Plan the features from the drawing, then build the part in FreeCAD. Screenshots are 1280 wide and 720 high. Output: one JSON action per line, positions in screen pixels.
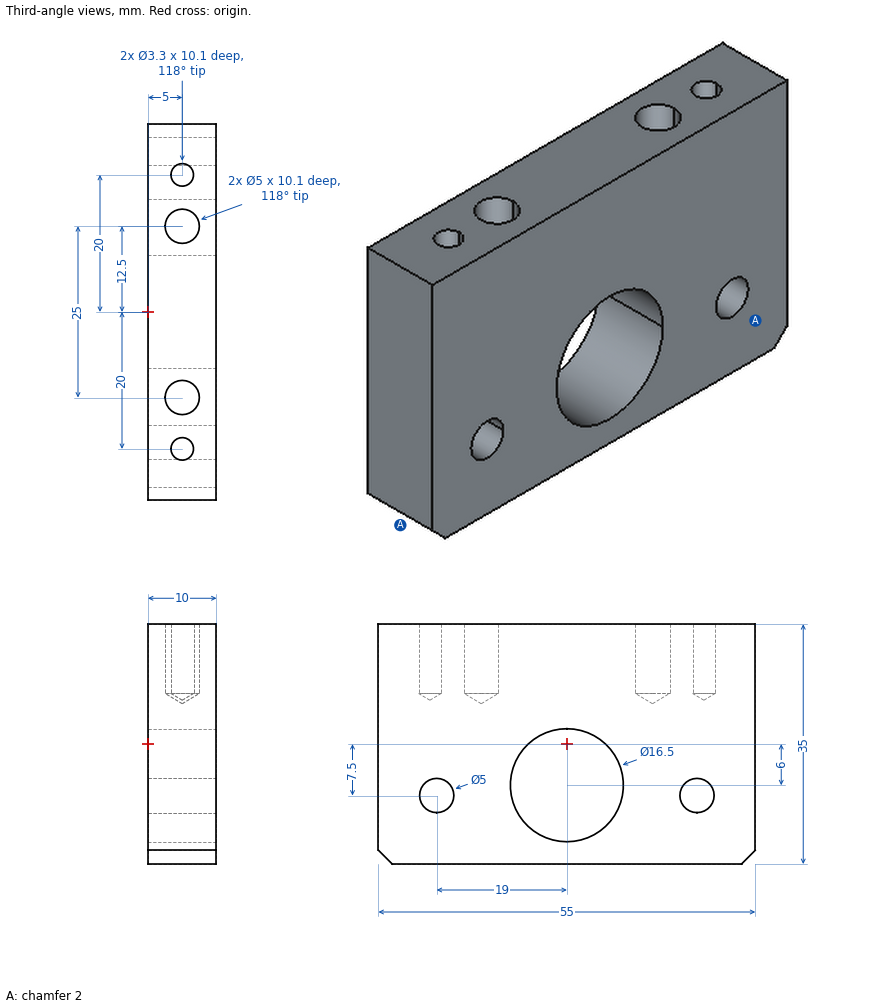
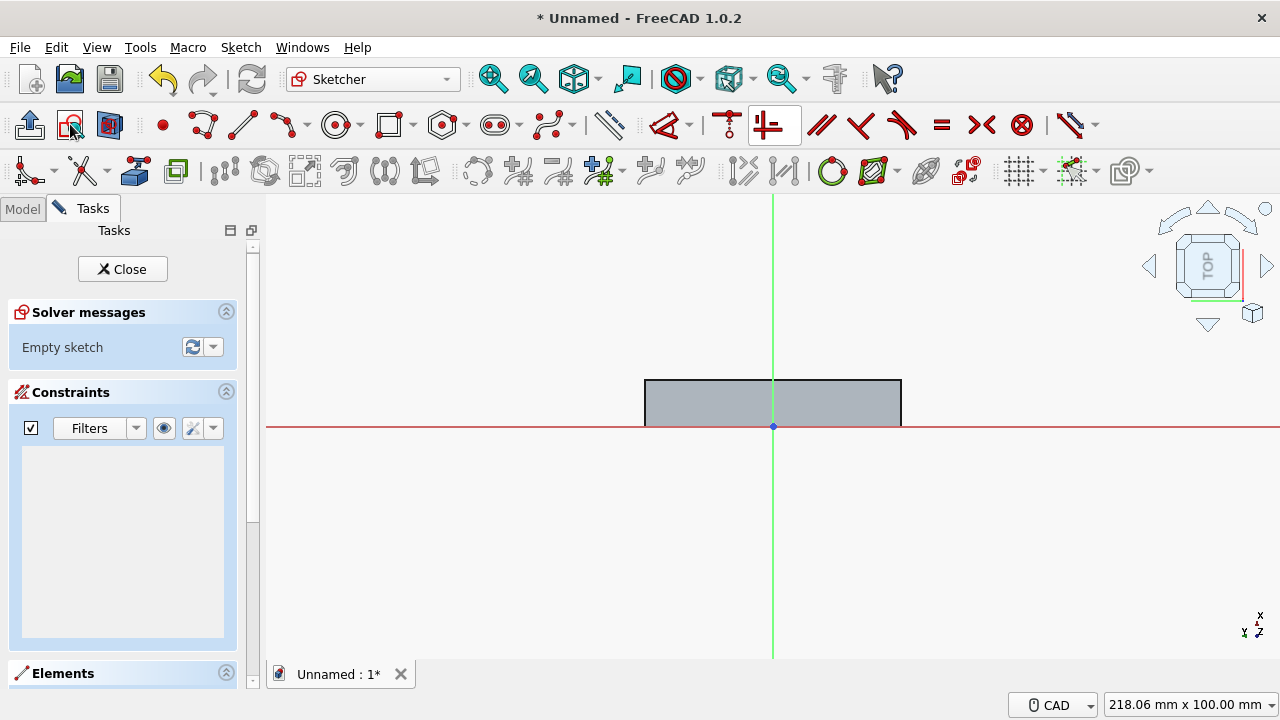
{"action": "scroll", "coordinate": [813, 402], "scroll_direction": "up", "scroll_amount": 5}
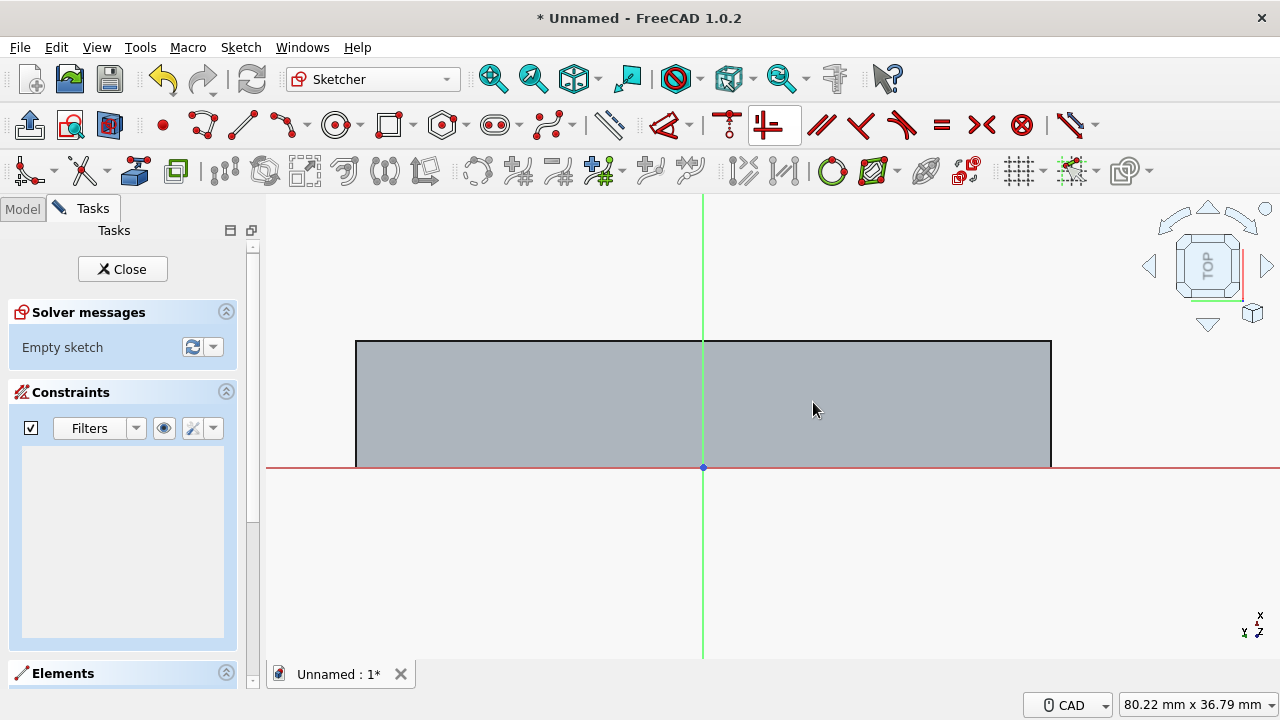
{"action": "left_click", "coordinate": [336, 126]}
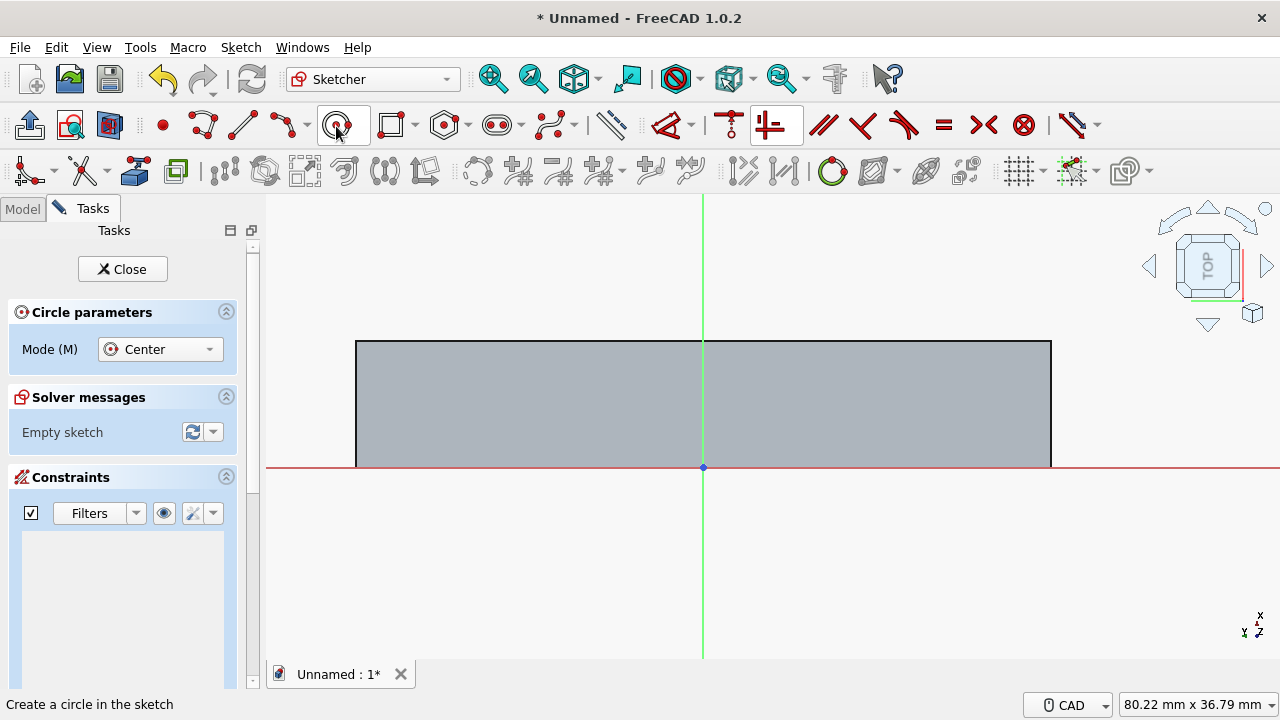
{"action": "left_click", "coordinate": [451, 405]}
{"action": "mouse_move", "coordinate": [465, 390]}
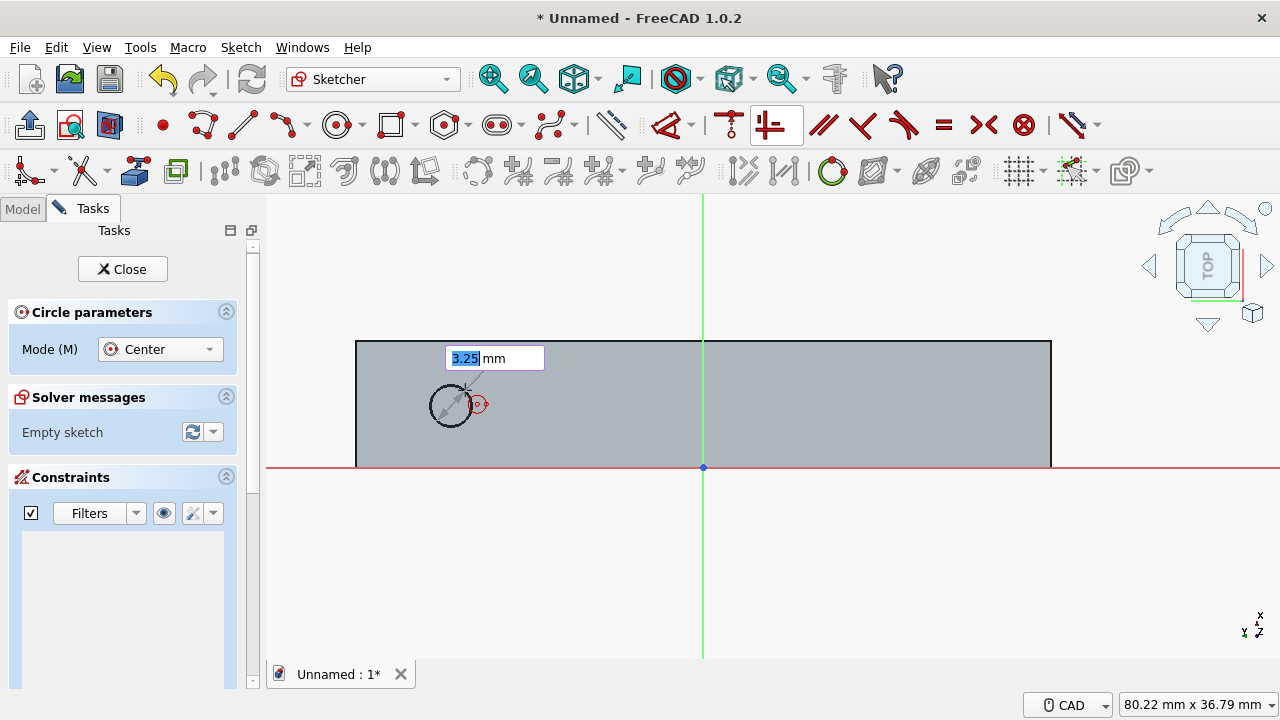
{"action": "type", "text": "3.3"}
{"action": "key", "text": "Return"}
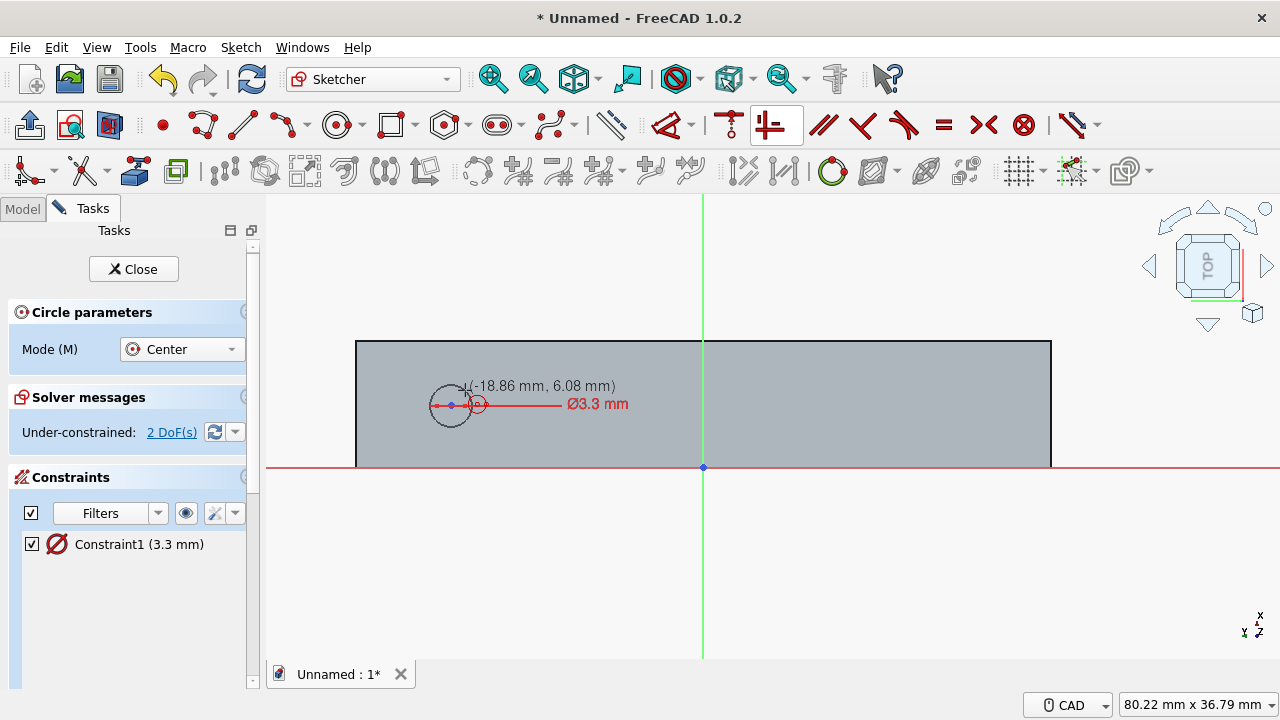
{"action": "left_click", "coordinate": [956, 405]}
{"action": "mouse_move", "coordinate": [971, 390]}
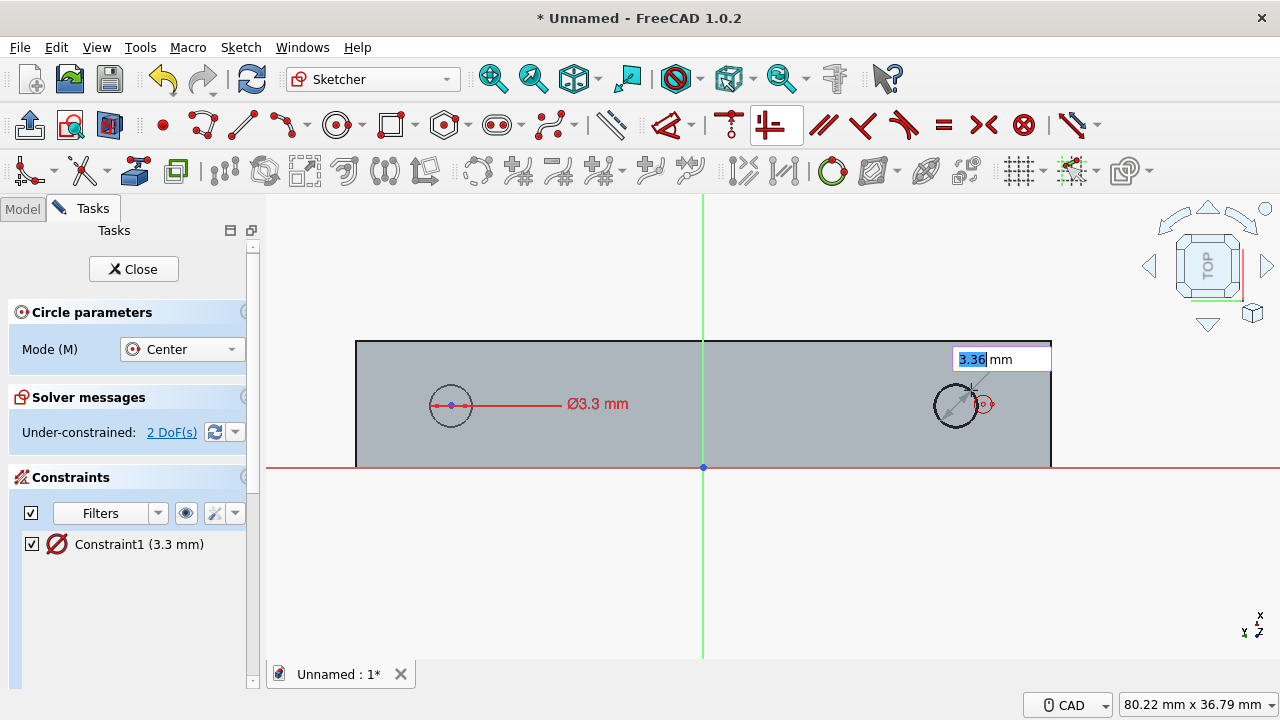
{"action": "type", "text": "3.3"}
{"action": "key", "text": "Return"}
{"action": "key", "text": "Escape"}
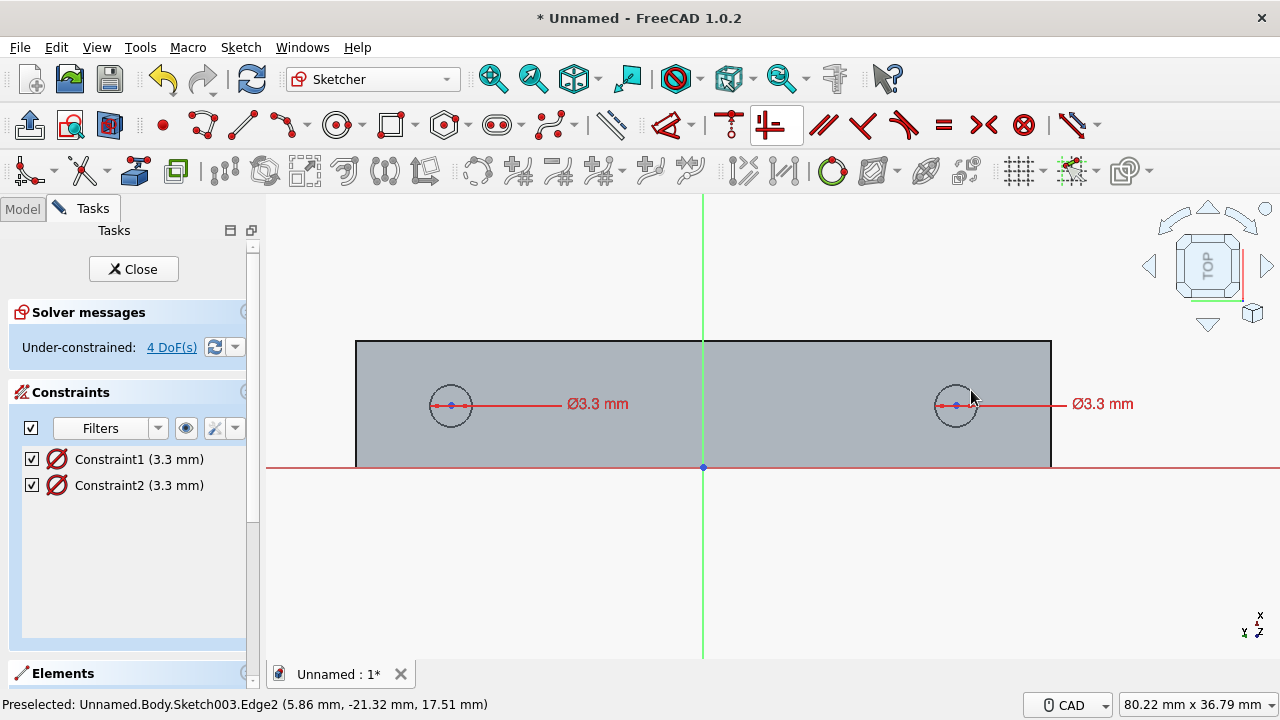
{"action": "left_click", "coordinate": [451, 406]}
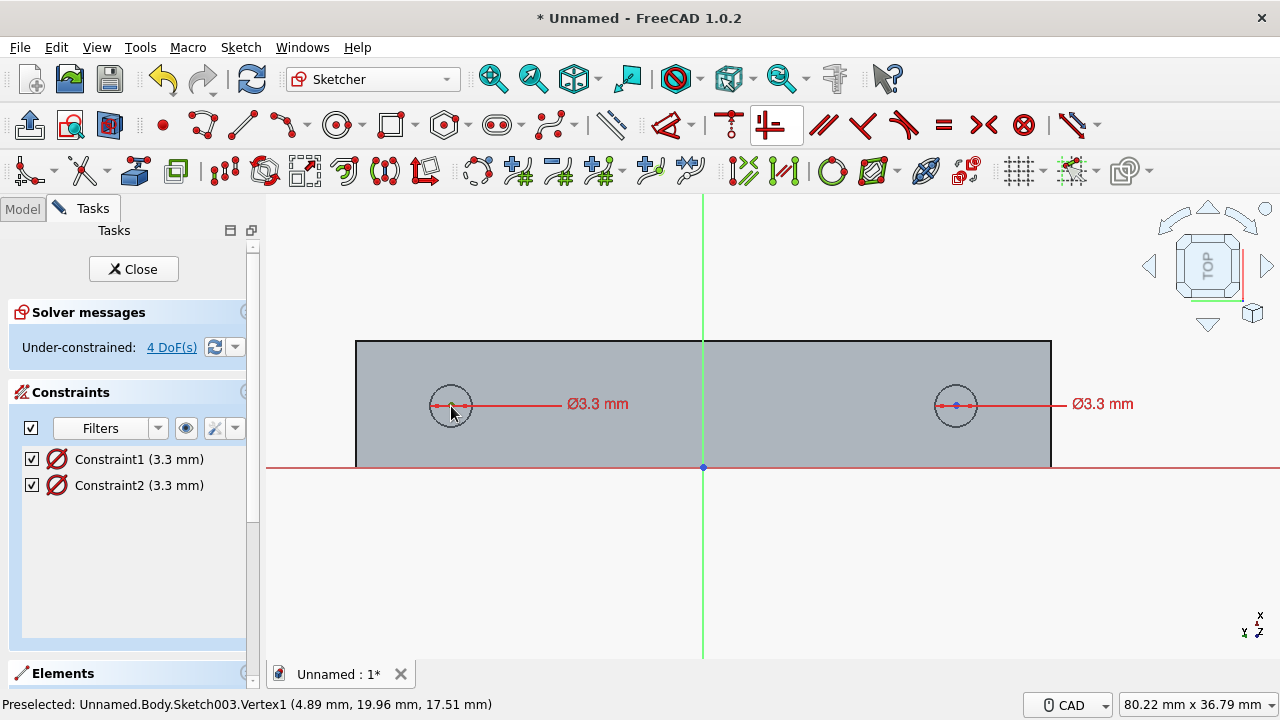
{"action": "left_click", "coordinate": [956, 406]}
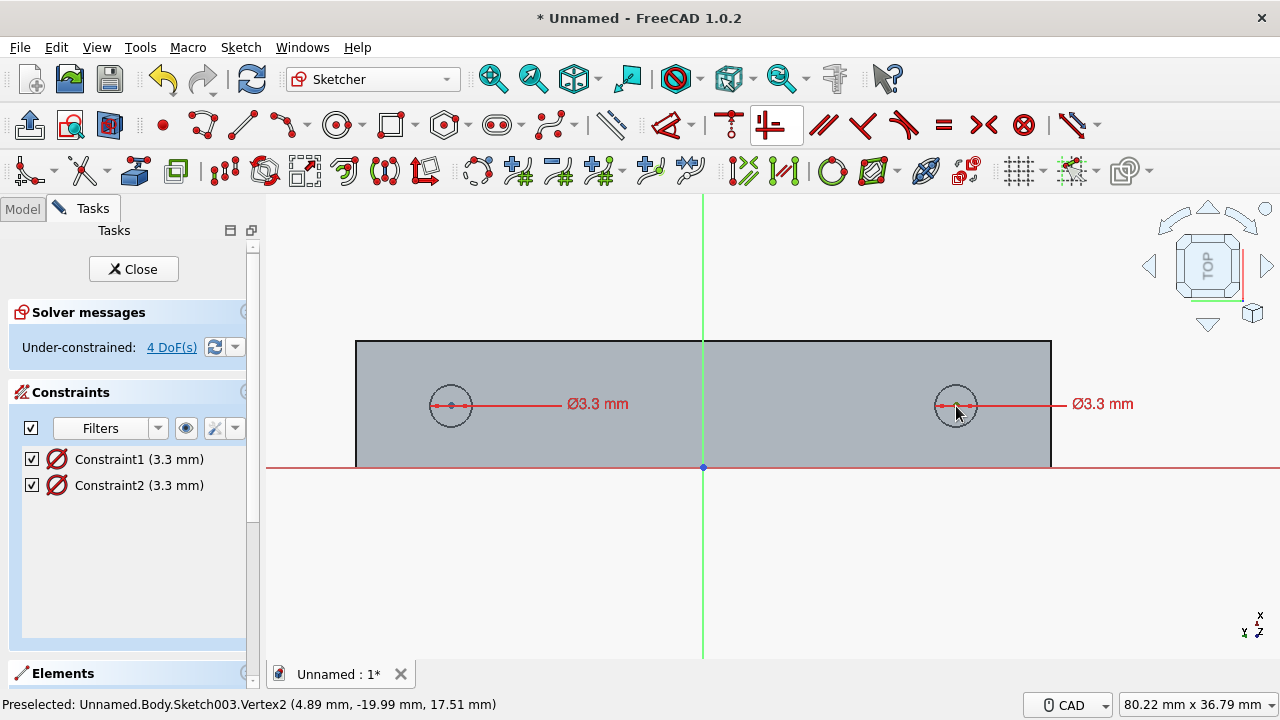
{"action": "left_click", "coordinate": [798, 126]}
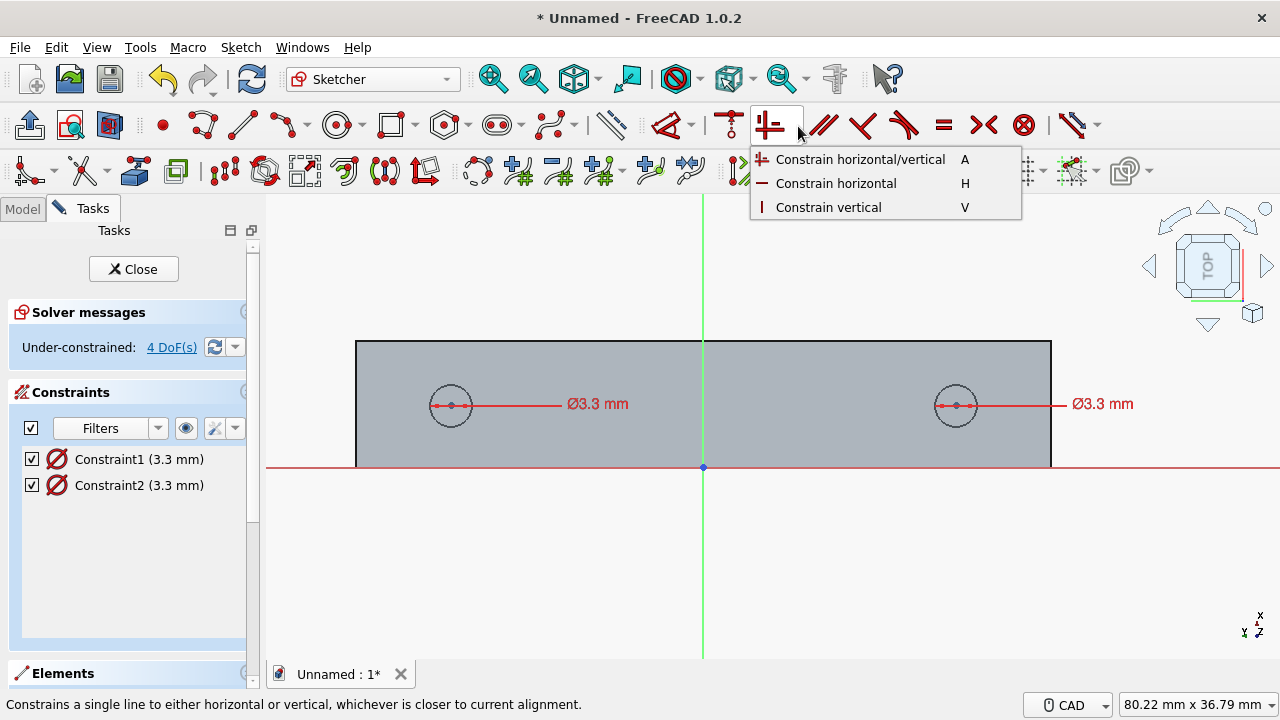
{"action": "left_click", "coordinate": [886, 183]}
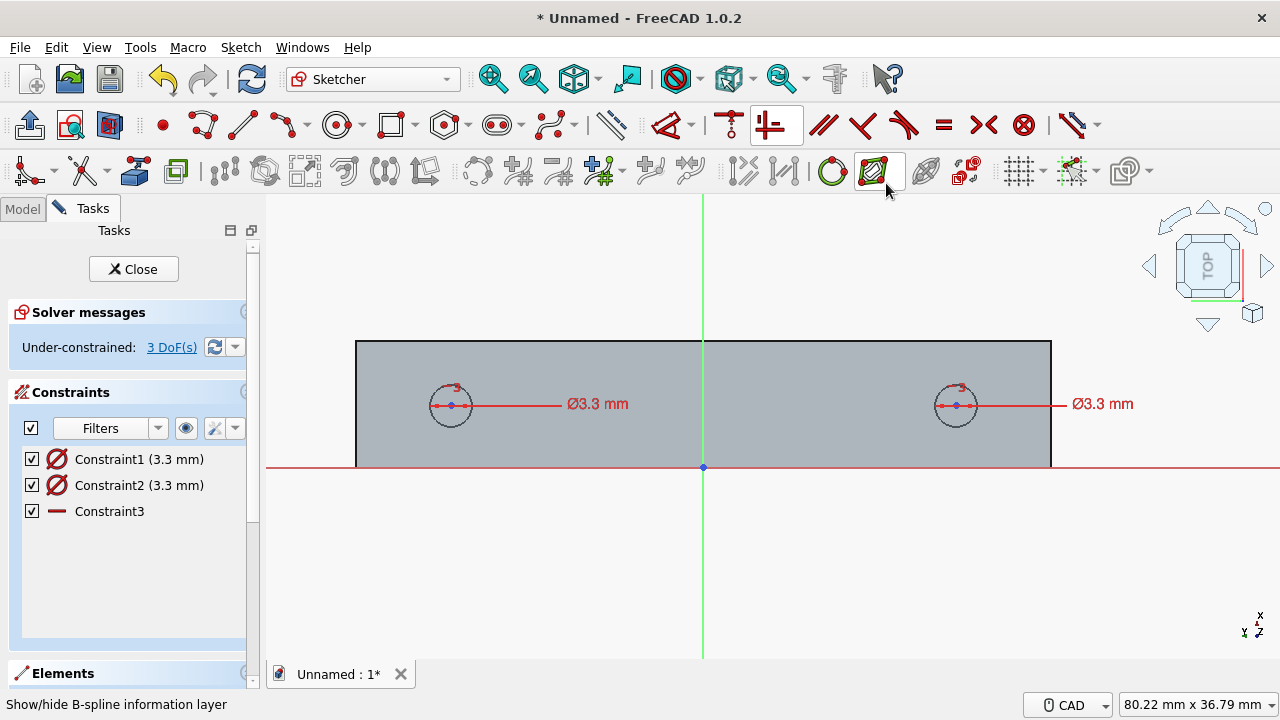
{"action": "left_click", "coordinate": [666, 126]}